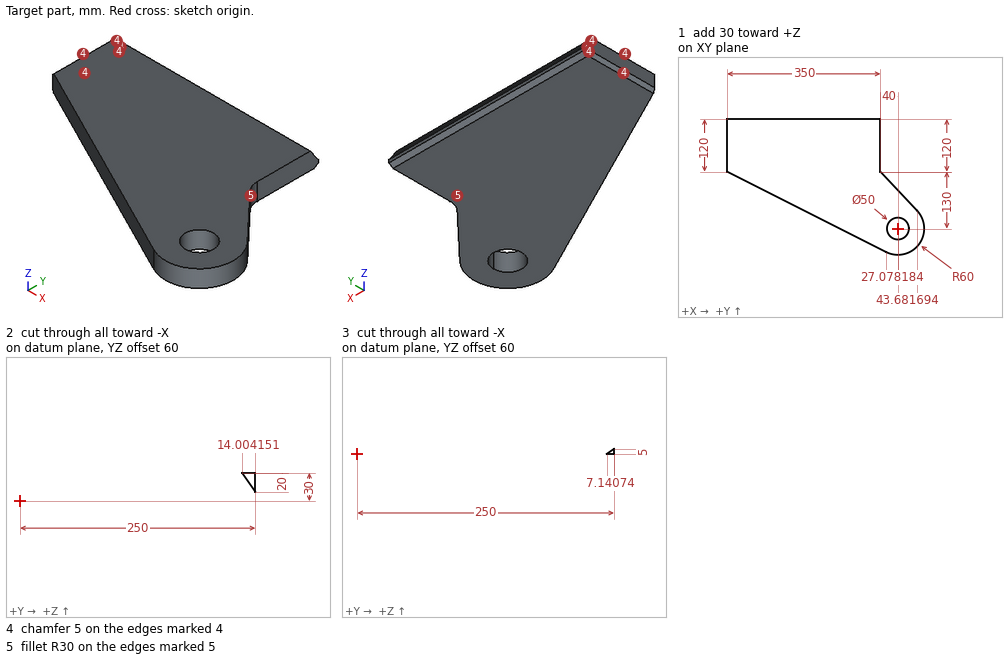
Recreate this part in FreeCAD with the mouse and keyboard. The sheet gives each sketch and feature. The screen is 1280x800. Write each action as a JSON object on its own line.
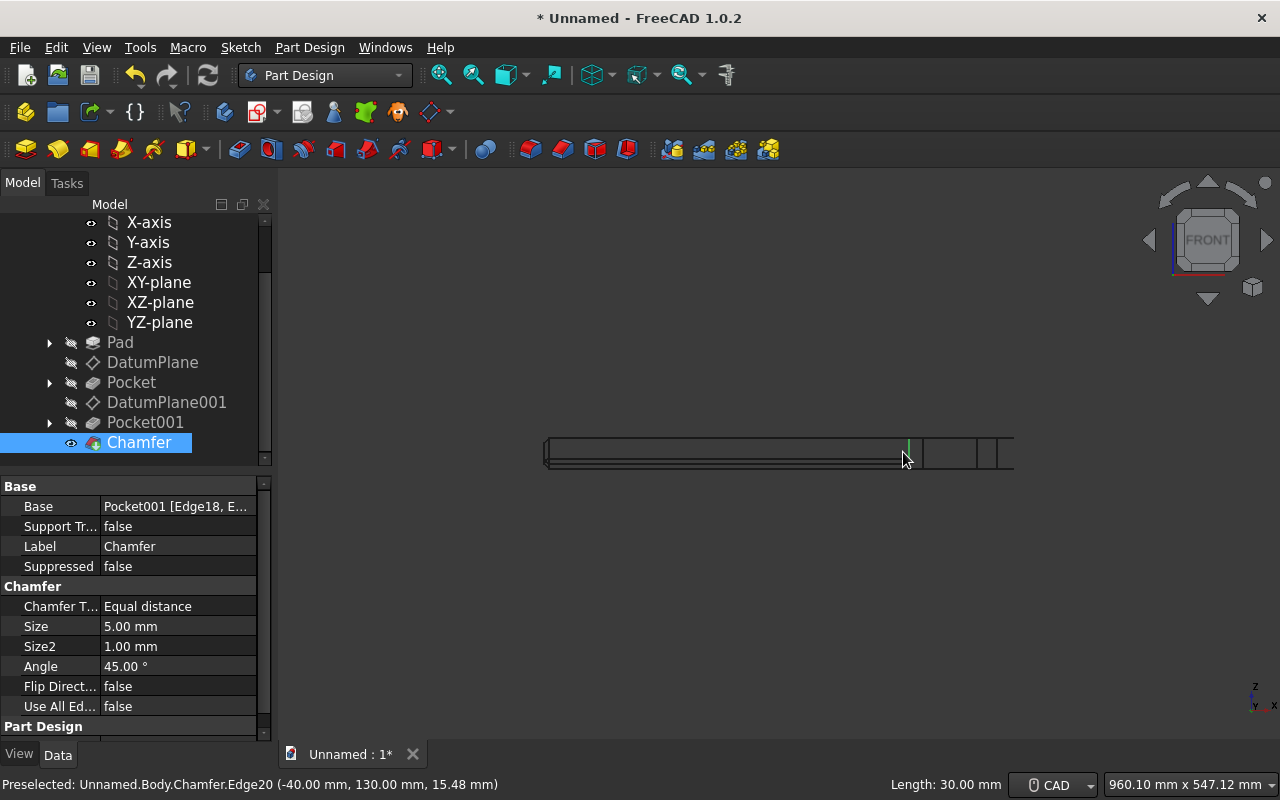
{"action": "key", "text": "v 1"}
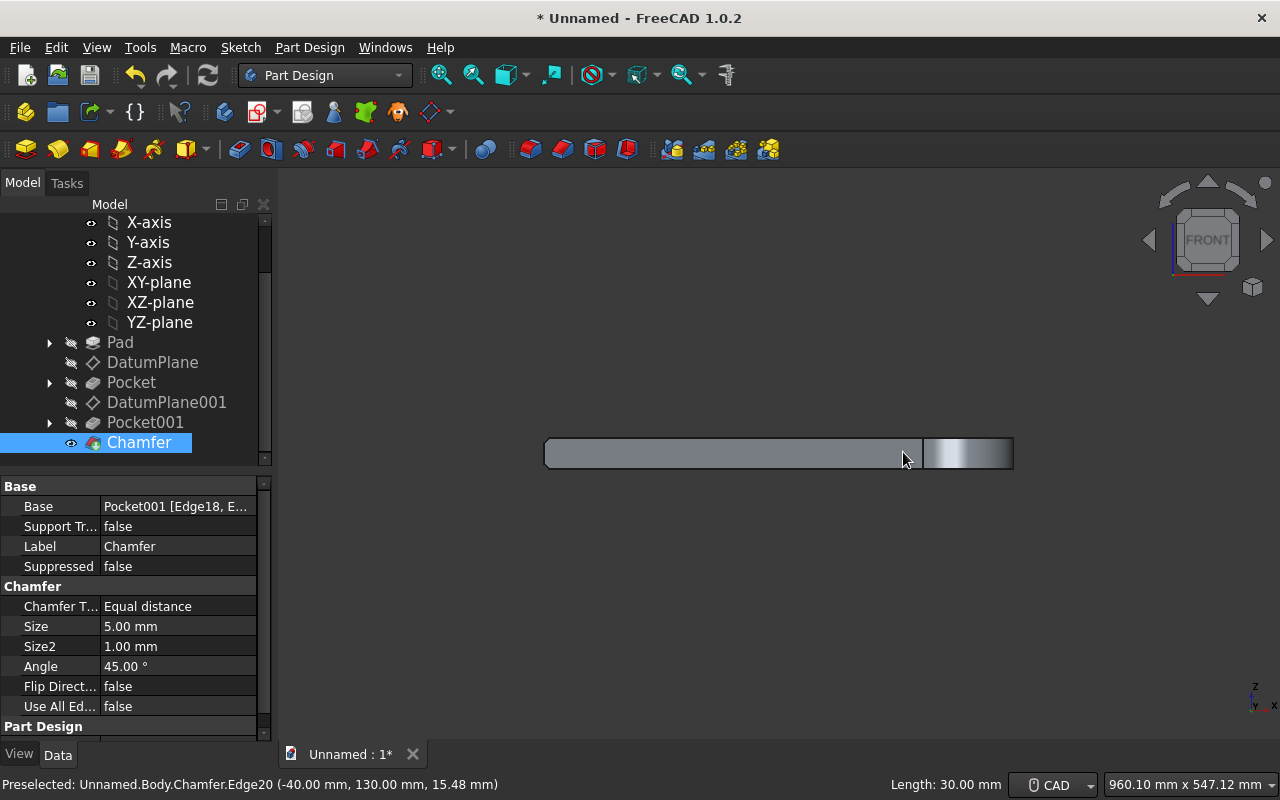
{"action": "left_click", "coordinate": [532, 150]}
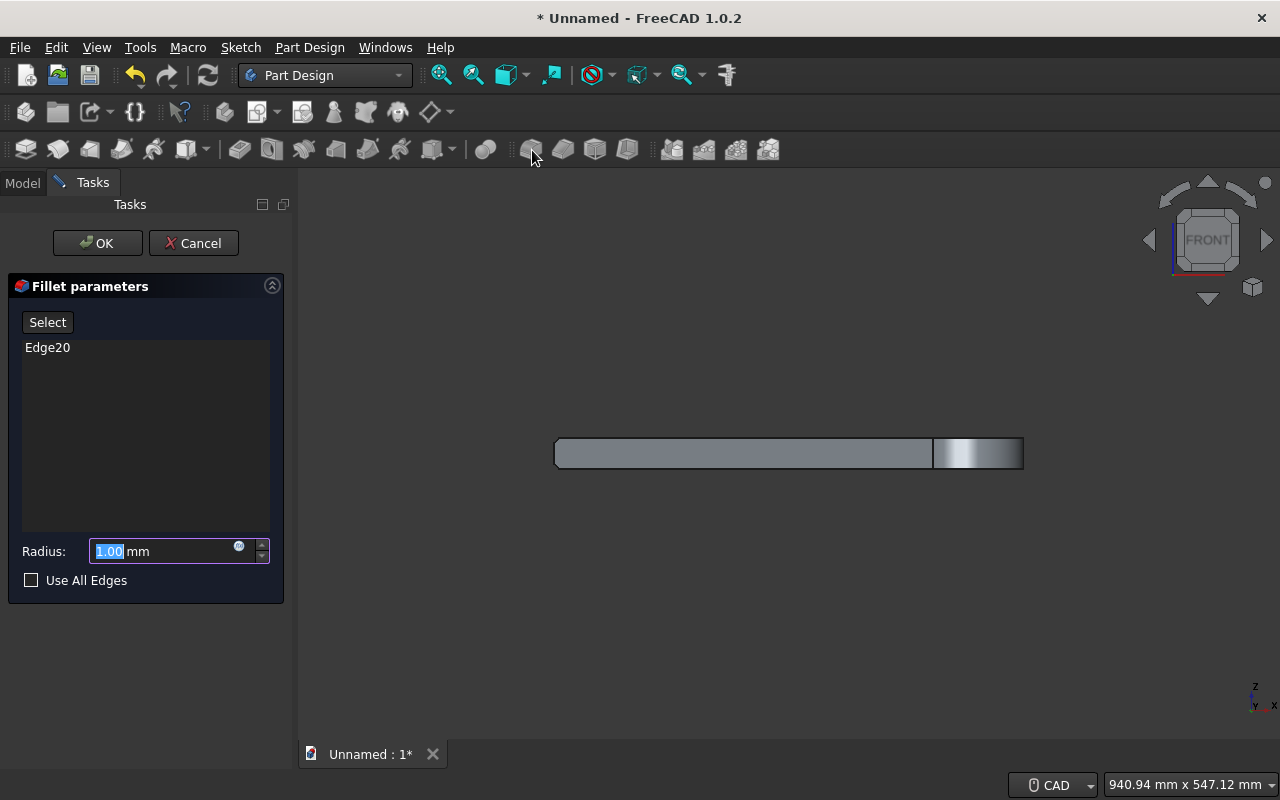
{"action": "type", "text": "30"}
{"action": "key", "text": "Tab"}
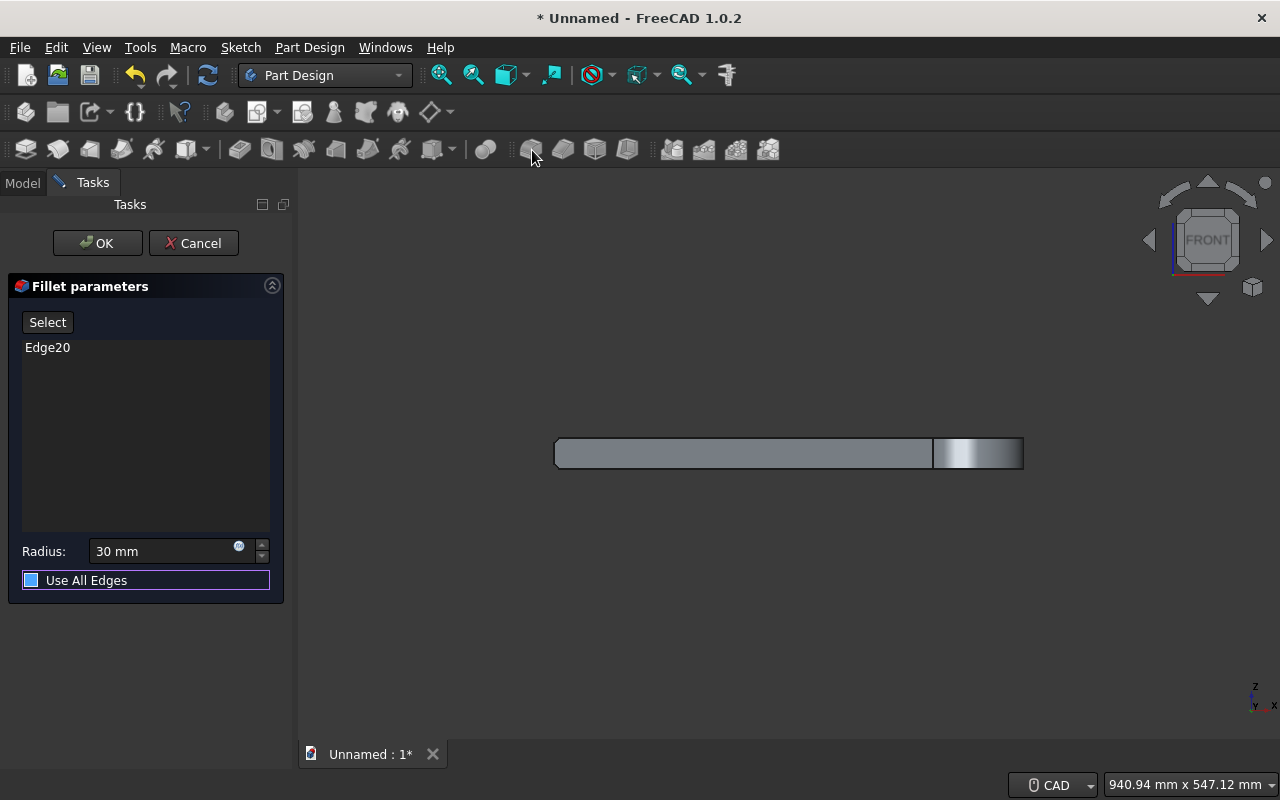
{"action": "left_click", "coordinate": [98, 243]}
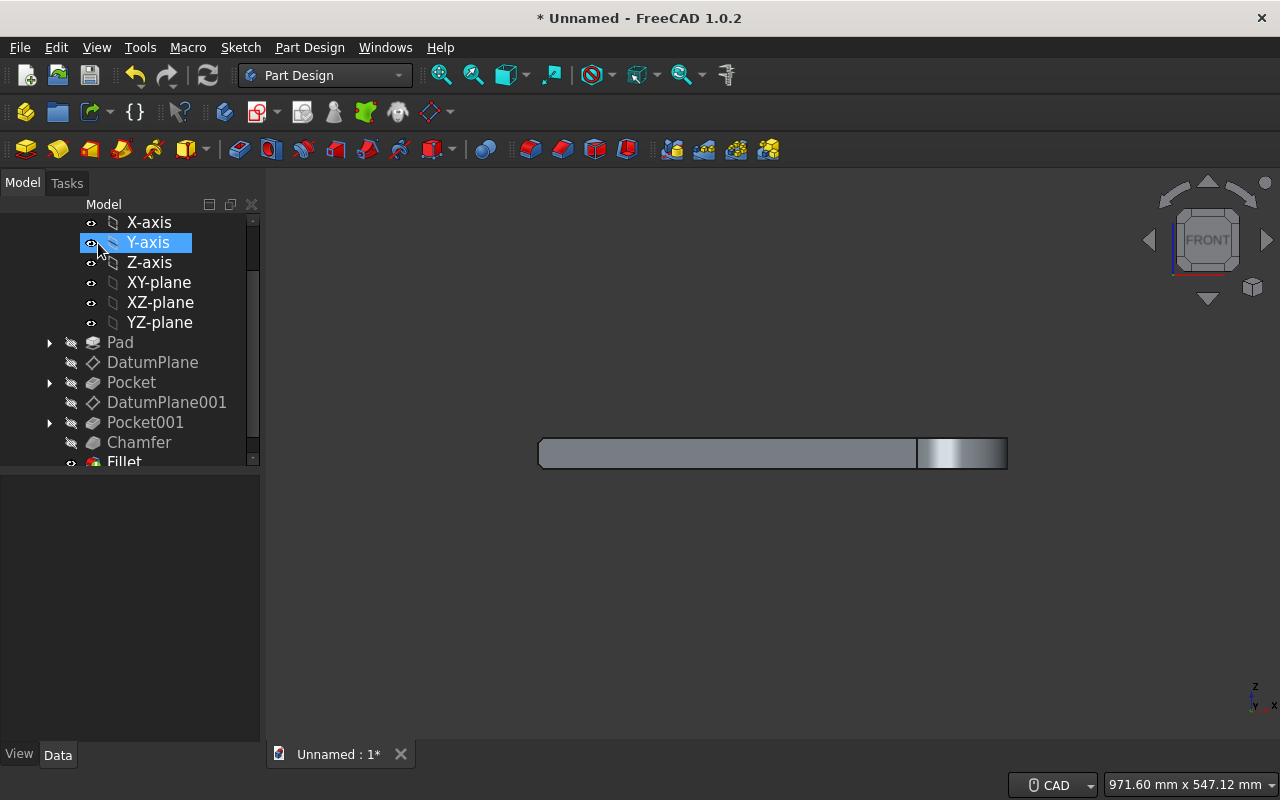
{"action": "key", "text": "0"}